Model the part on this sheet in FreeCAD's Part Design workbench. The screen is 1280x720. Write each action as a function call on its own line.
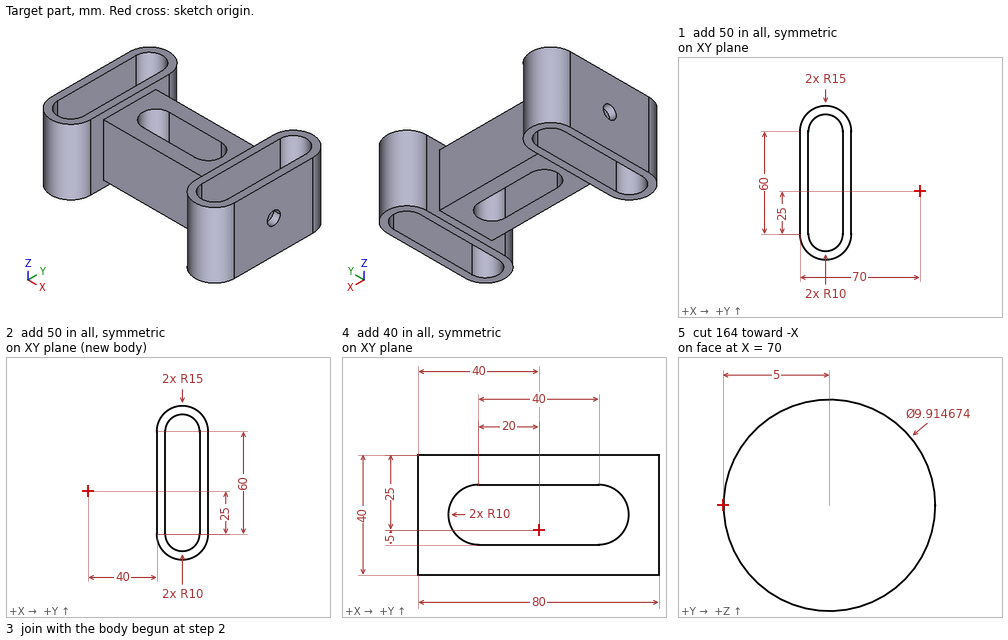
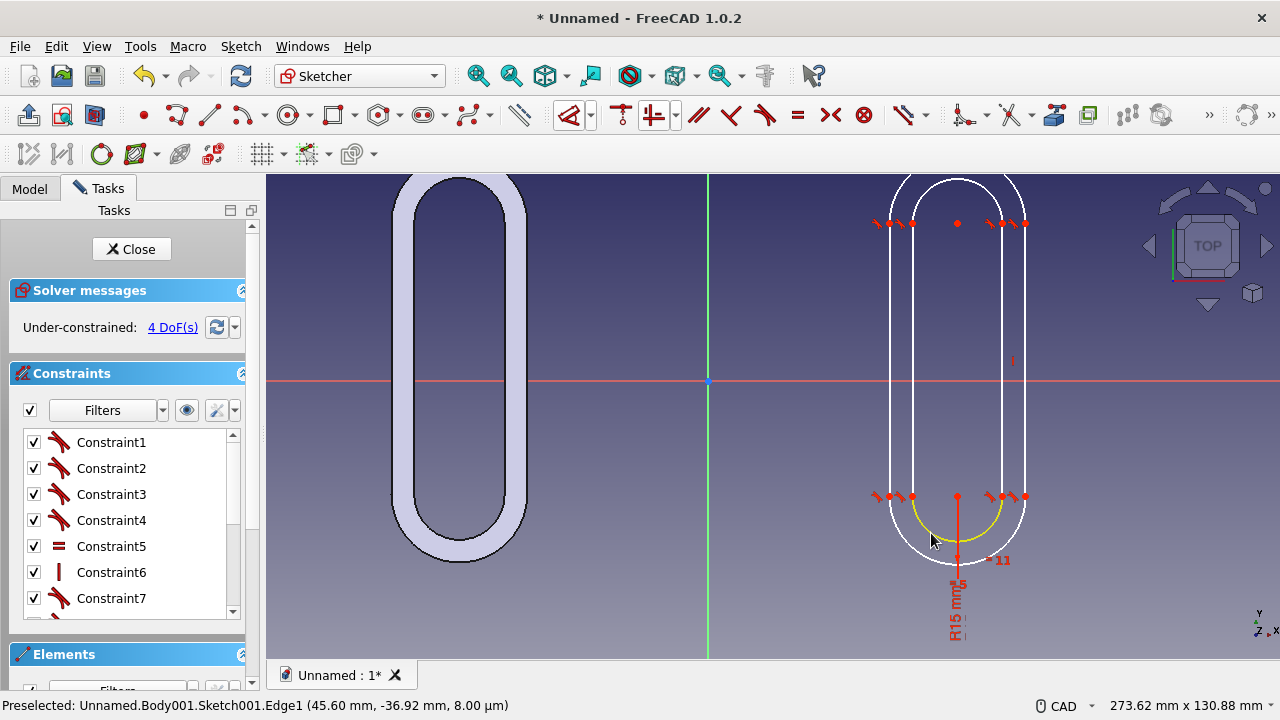
click(931, 533)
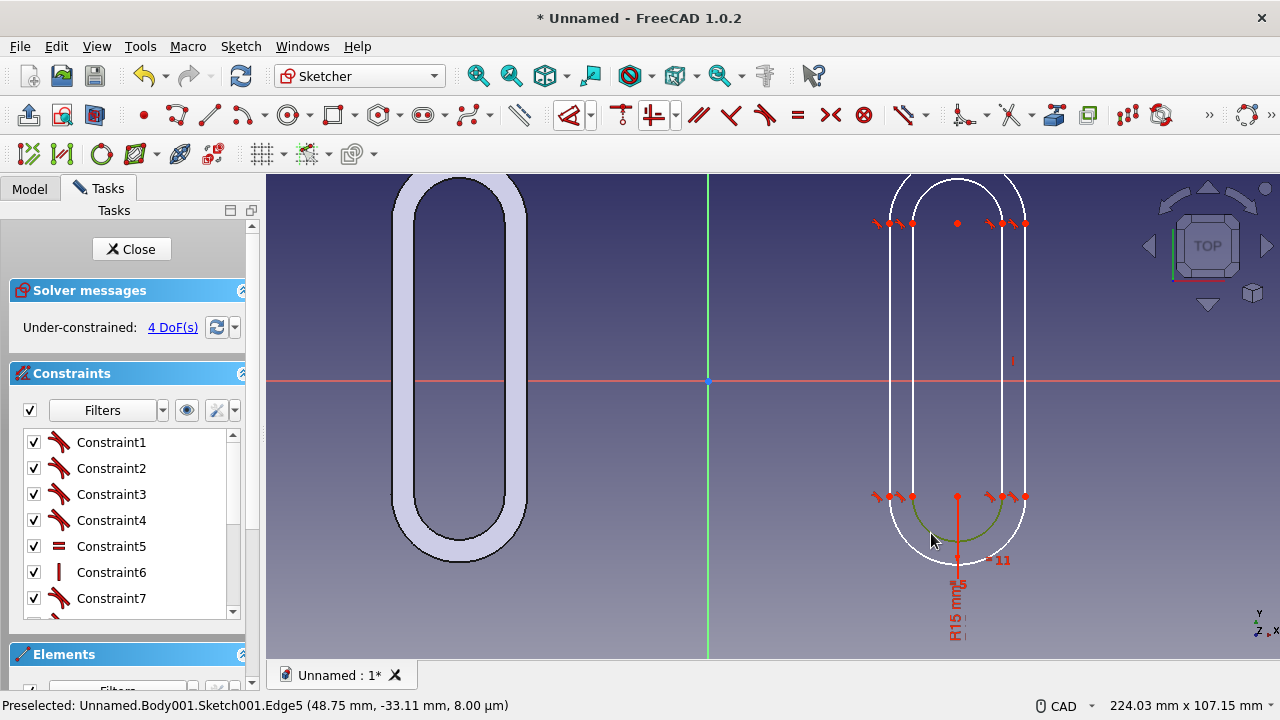
click(590, 116)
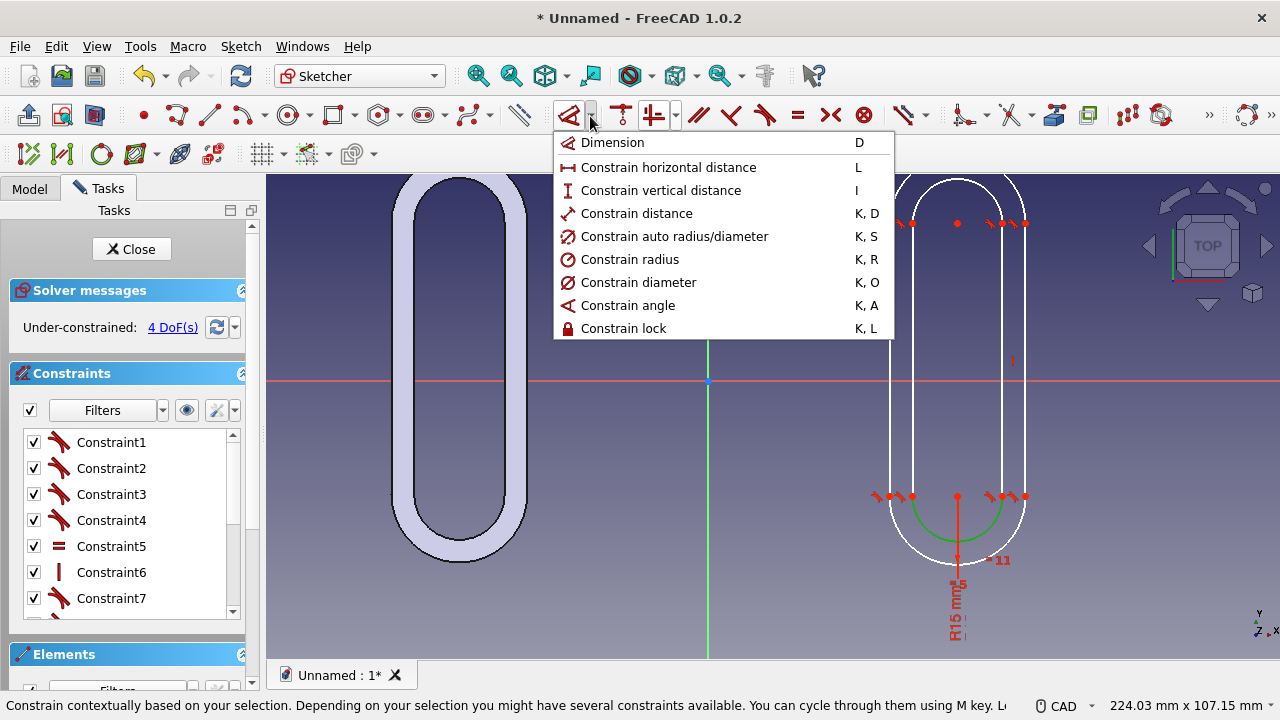
click(724, 260)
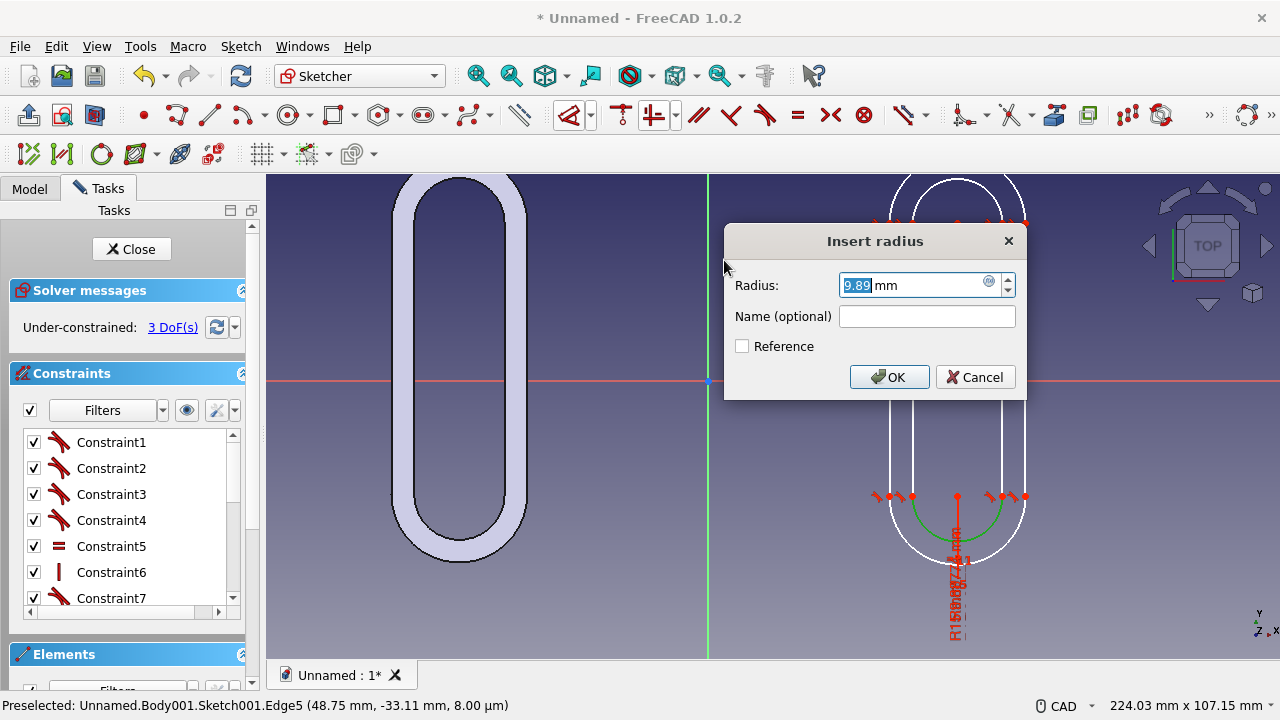
text(10)
key(Return)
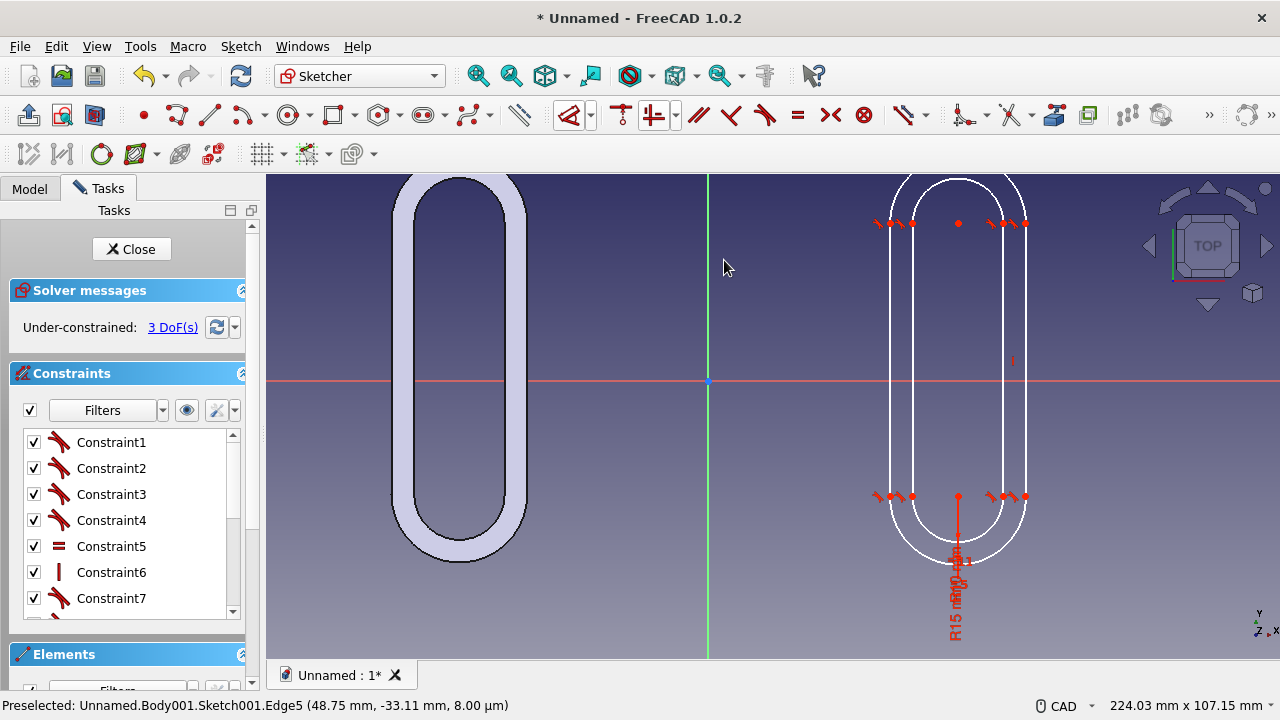
click(890, 415)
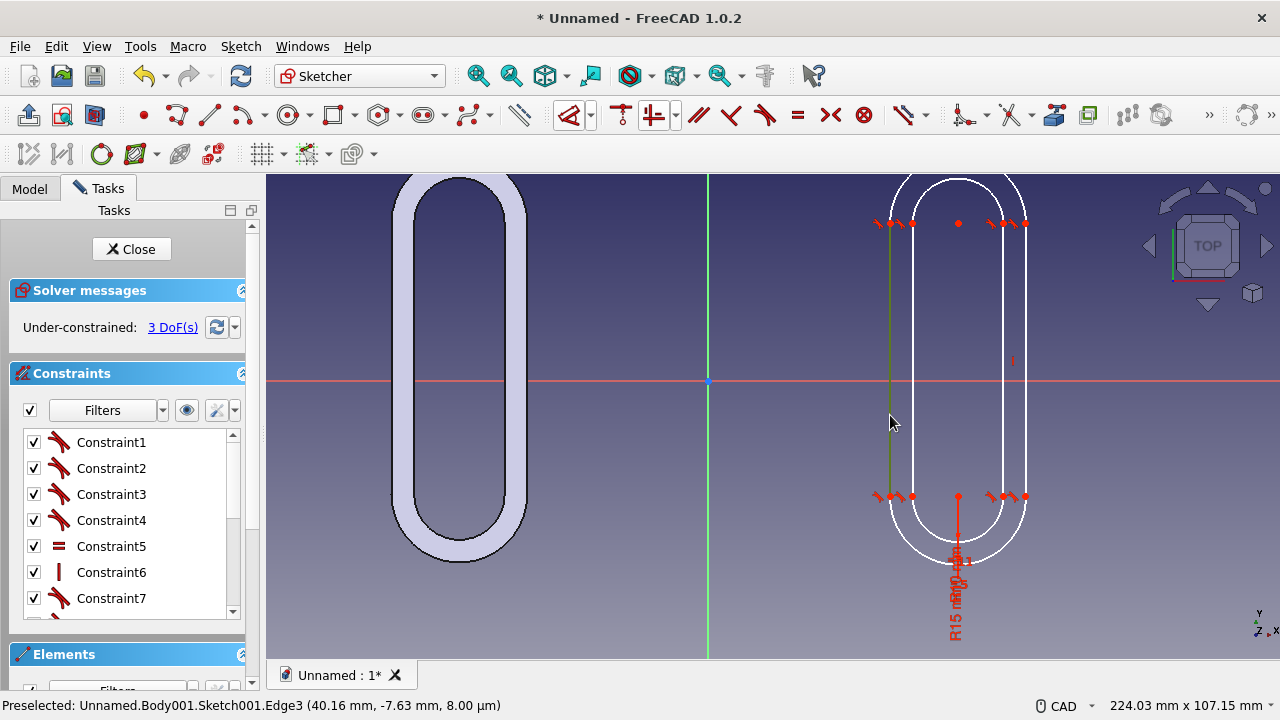
click(590, 116)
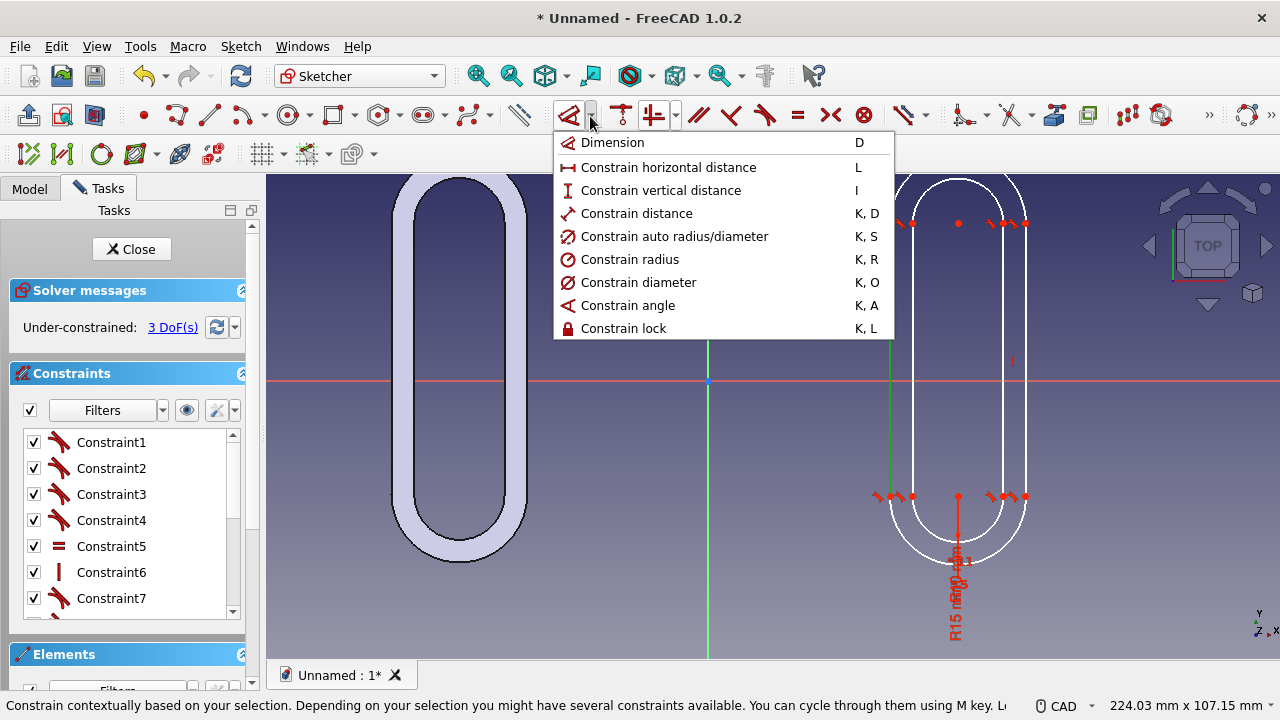
click(724, 190)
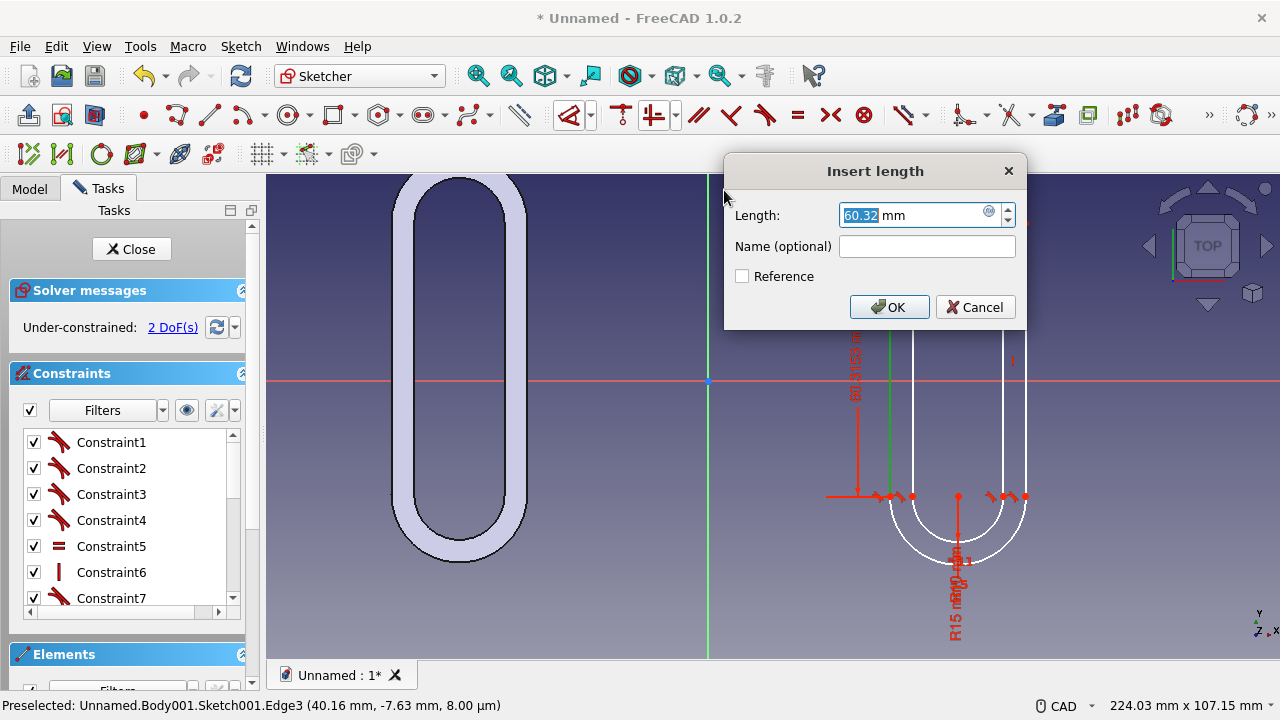
text(60)
key(Return)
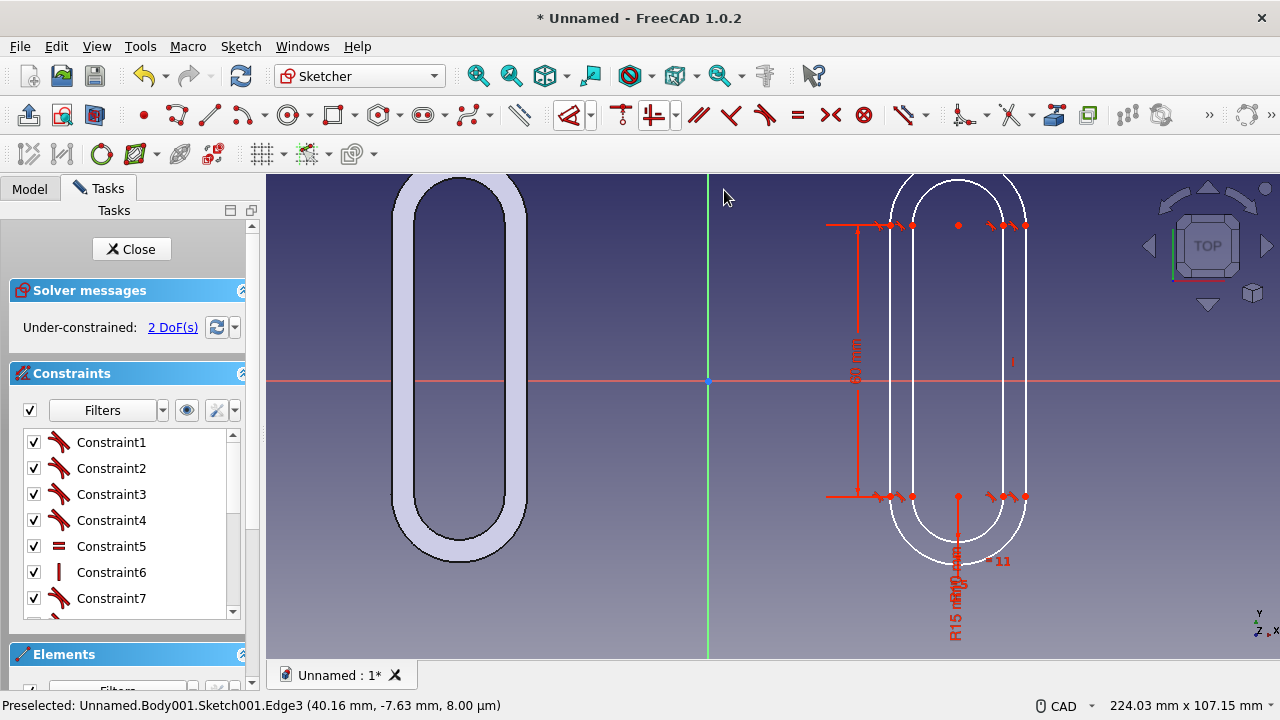
click(890, 497)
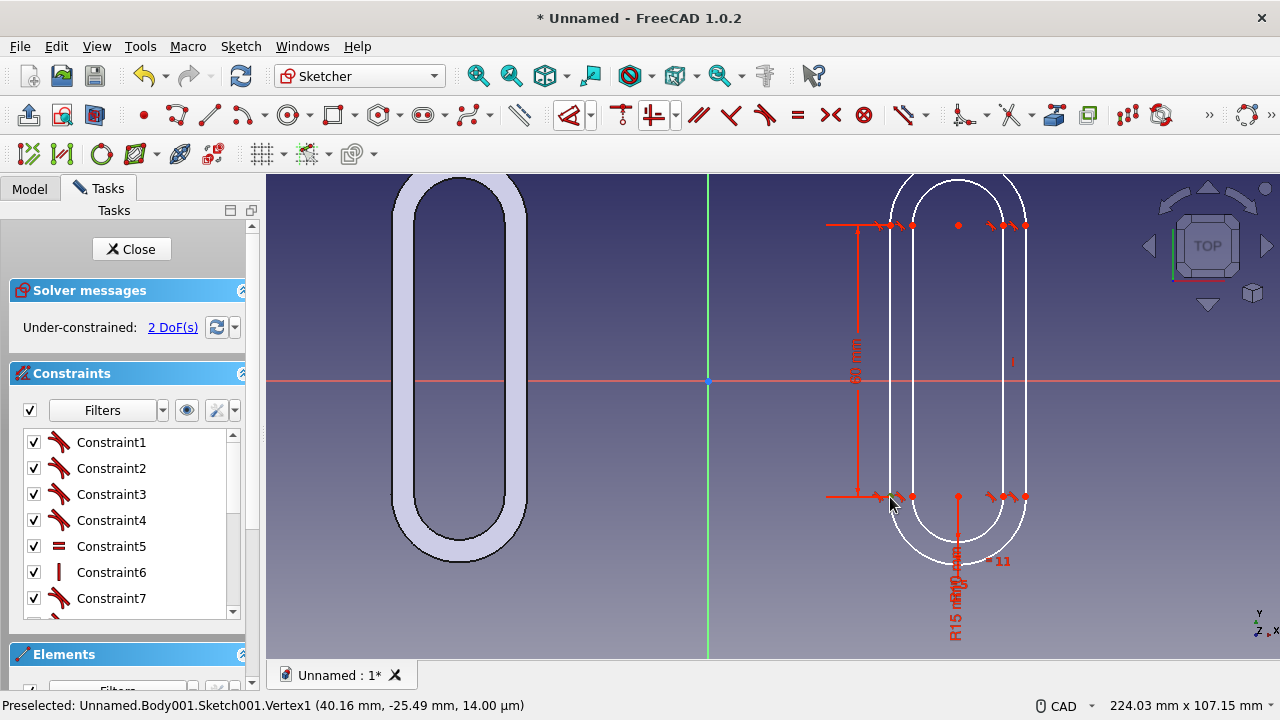
click(590, 116)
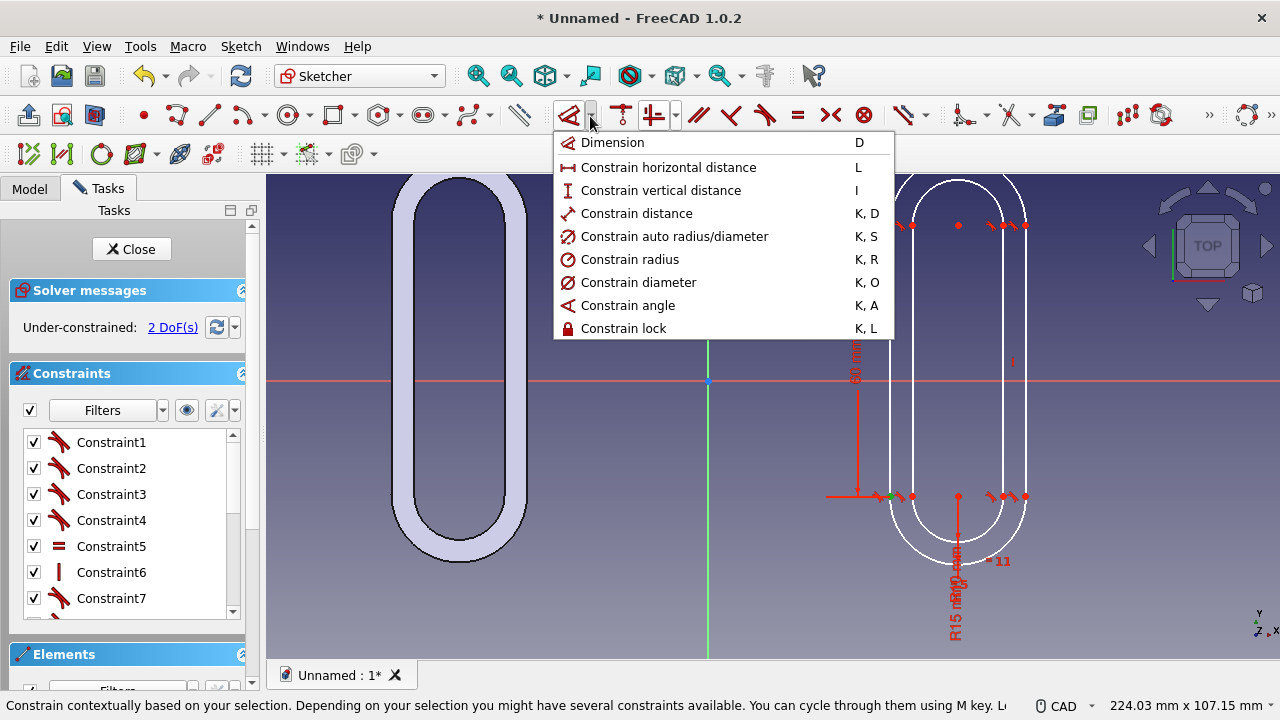
click(724, 168)